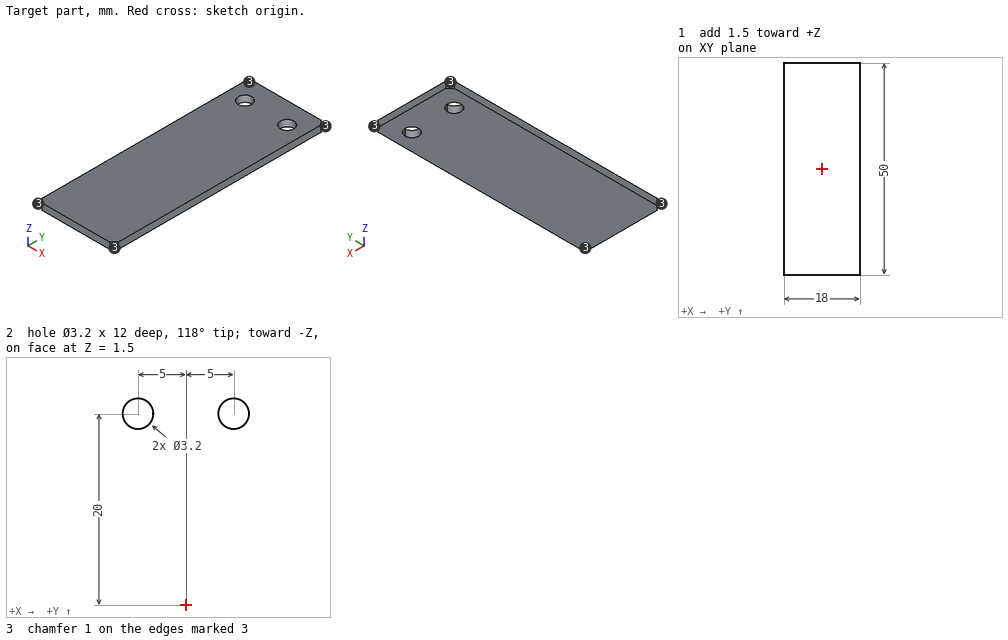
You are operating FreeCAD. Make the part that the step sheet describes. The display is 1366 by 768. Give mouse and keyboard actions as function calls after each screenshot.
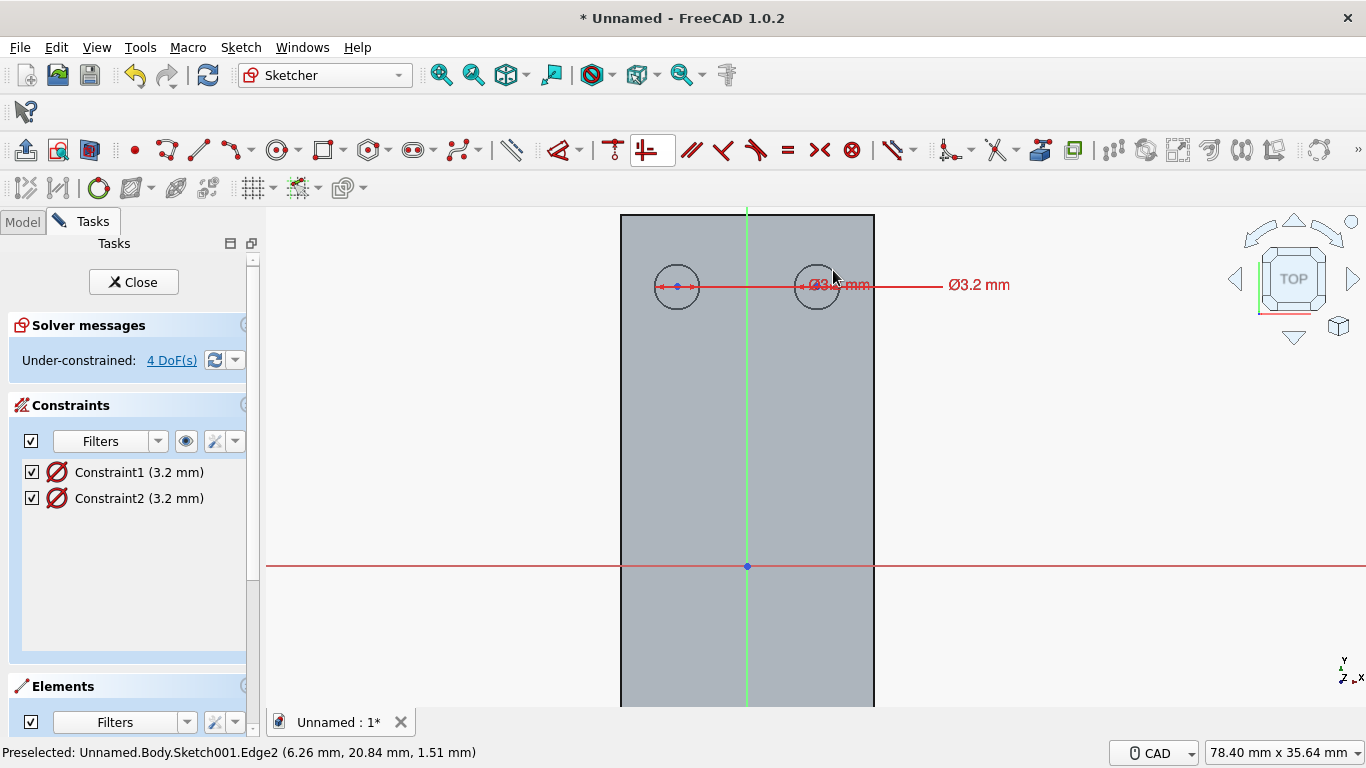
click(677, 287)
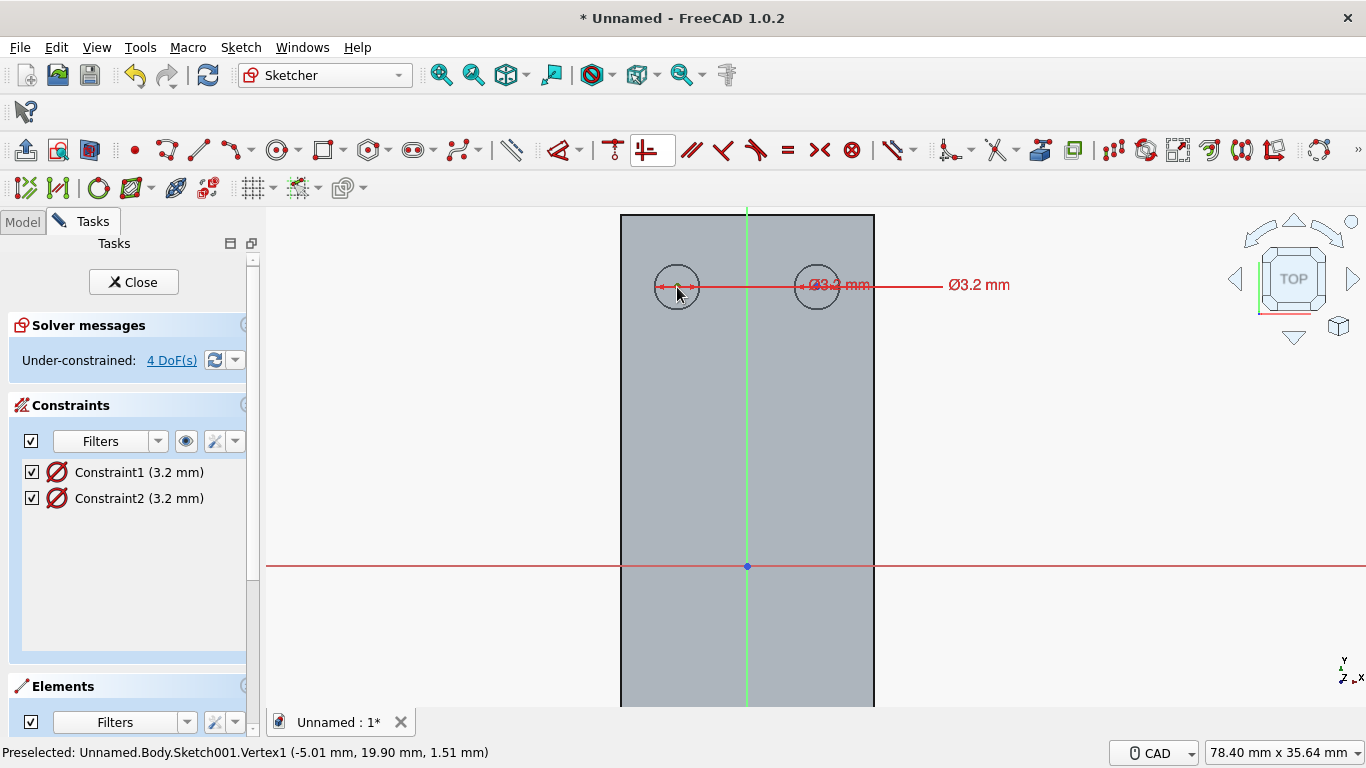
click(817, 287)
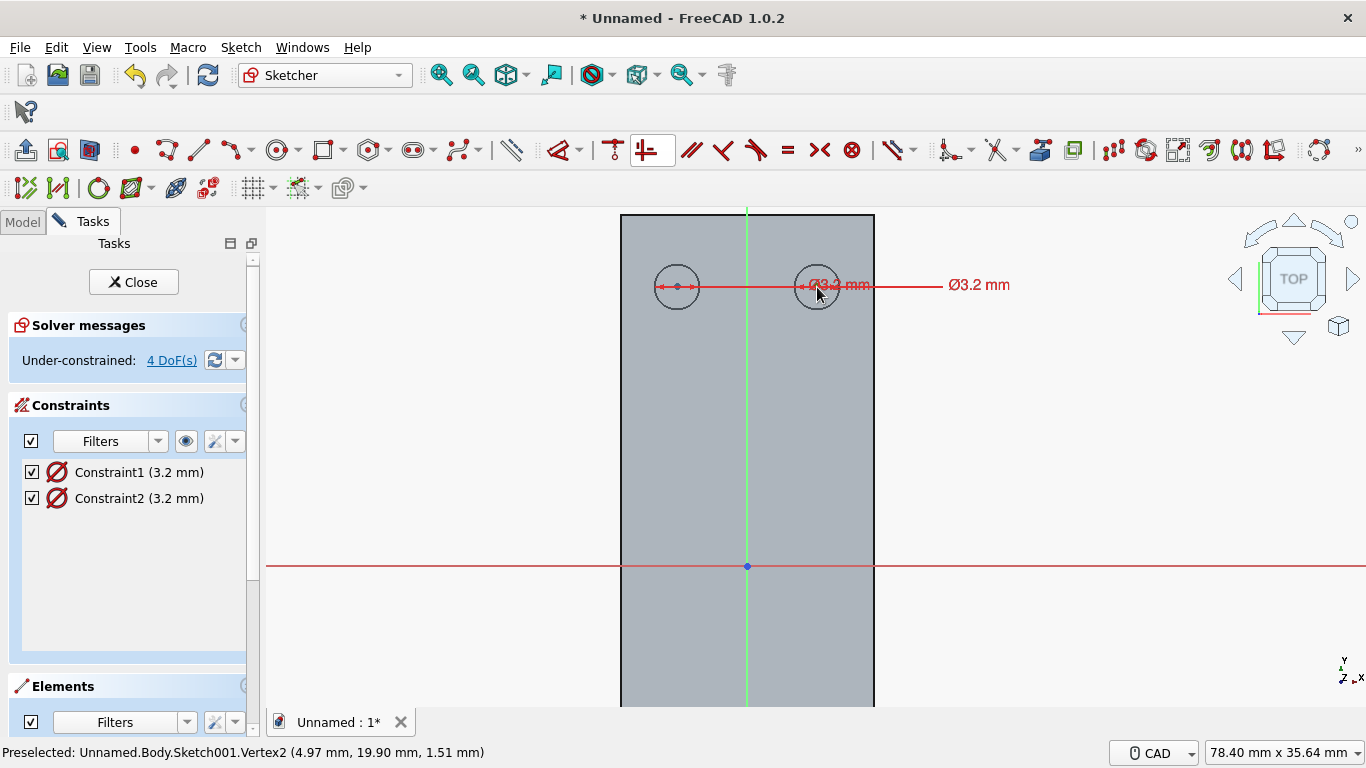
key(h)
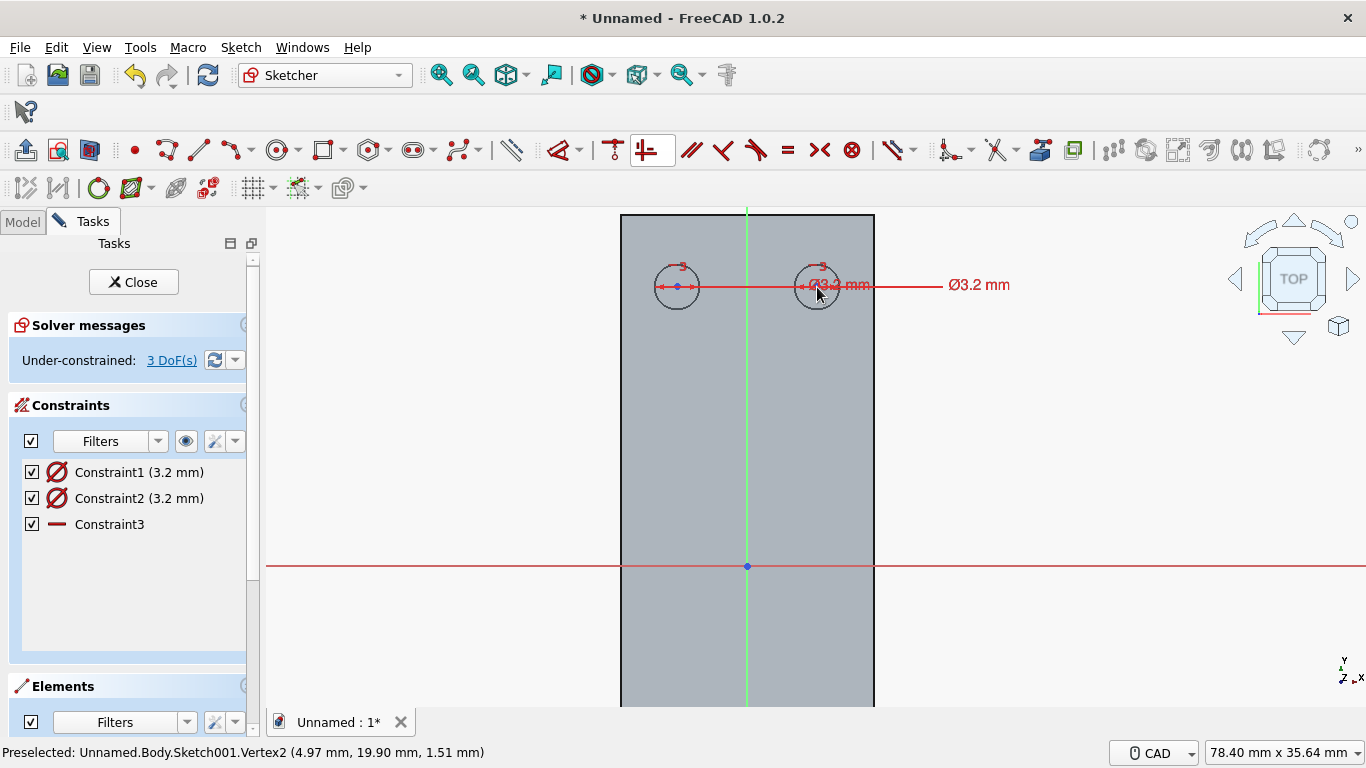
click(677, 287)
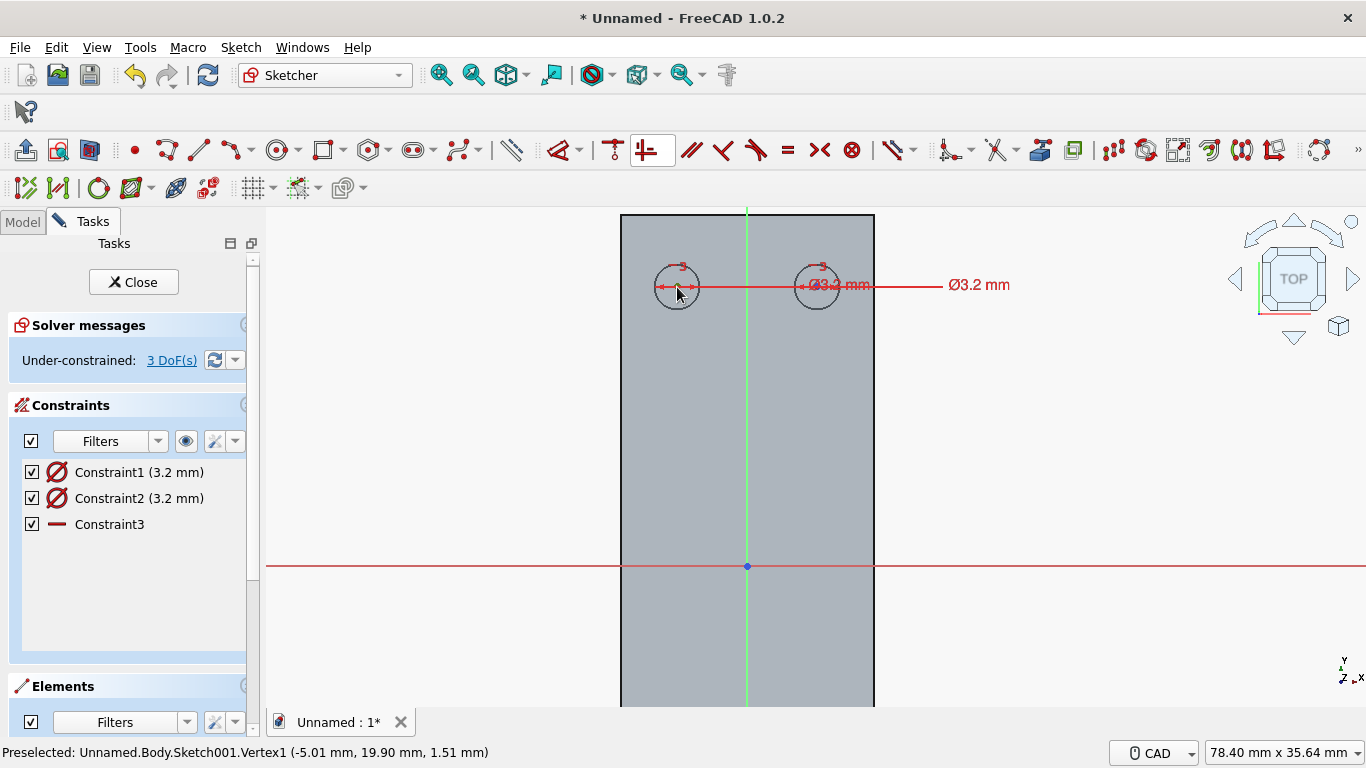
key(l)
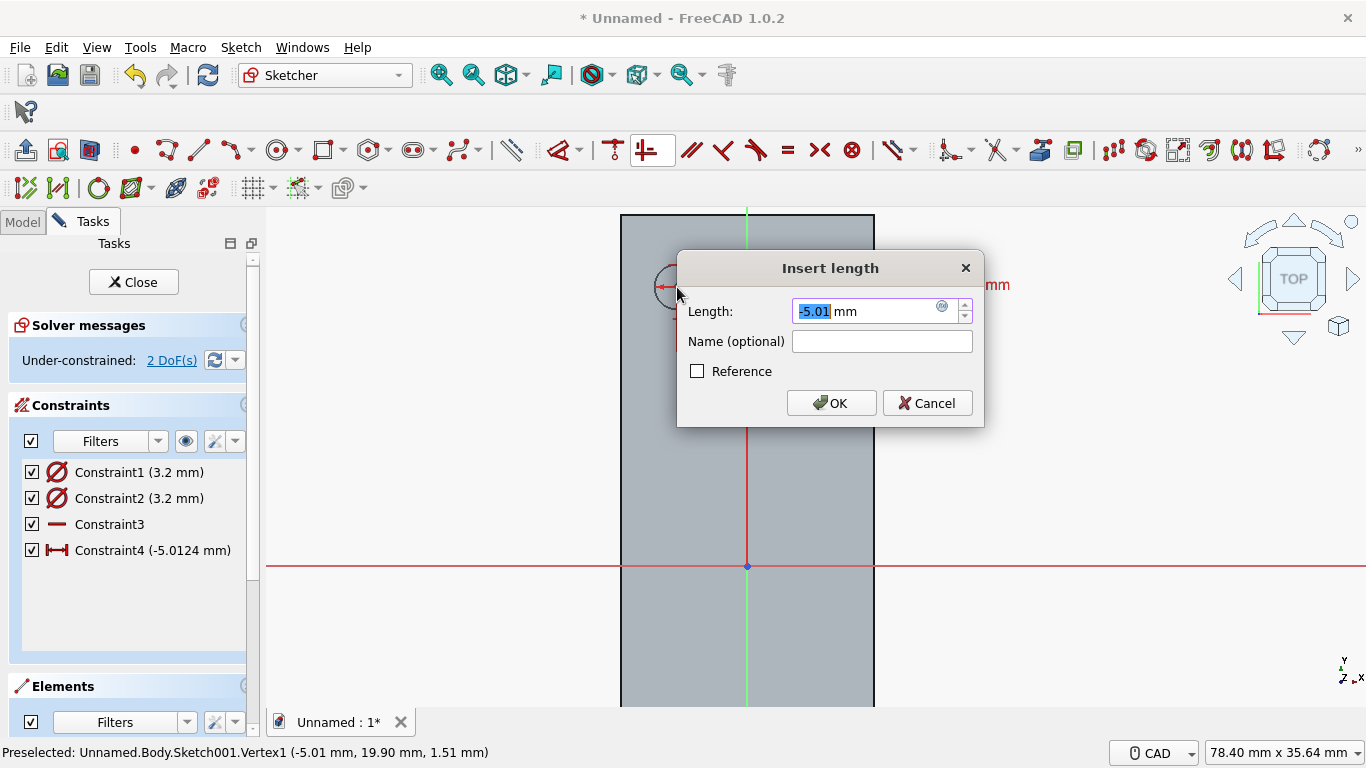
text(-5)
key(Return)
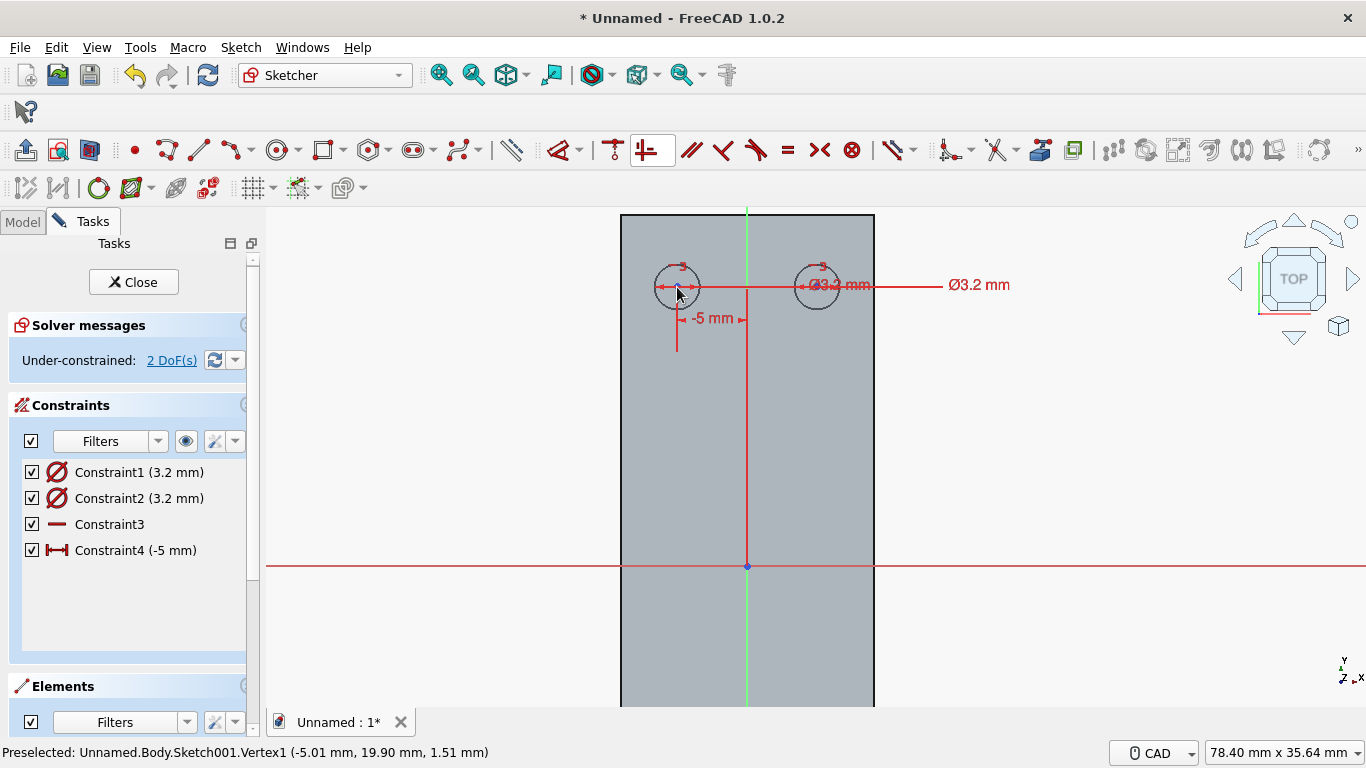
click(817, 287)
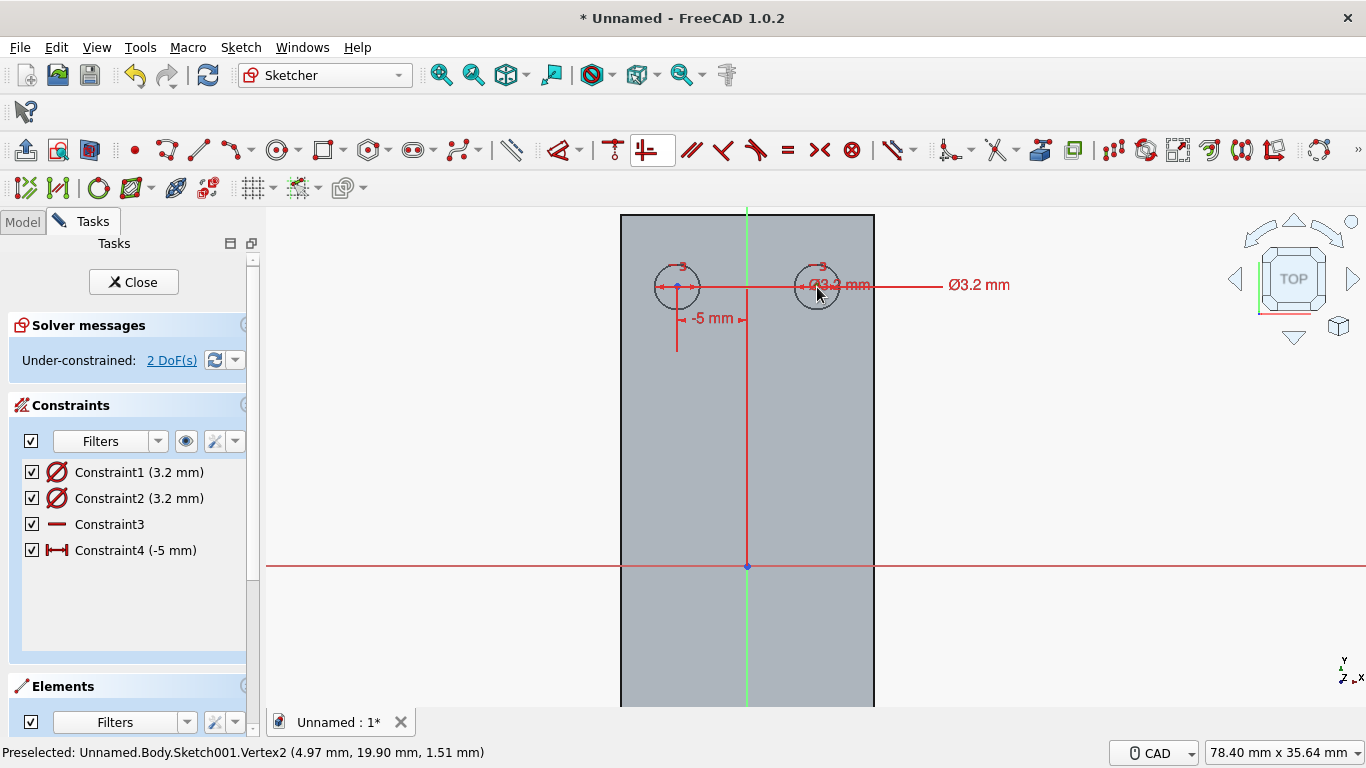
click(582, 150)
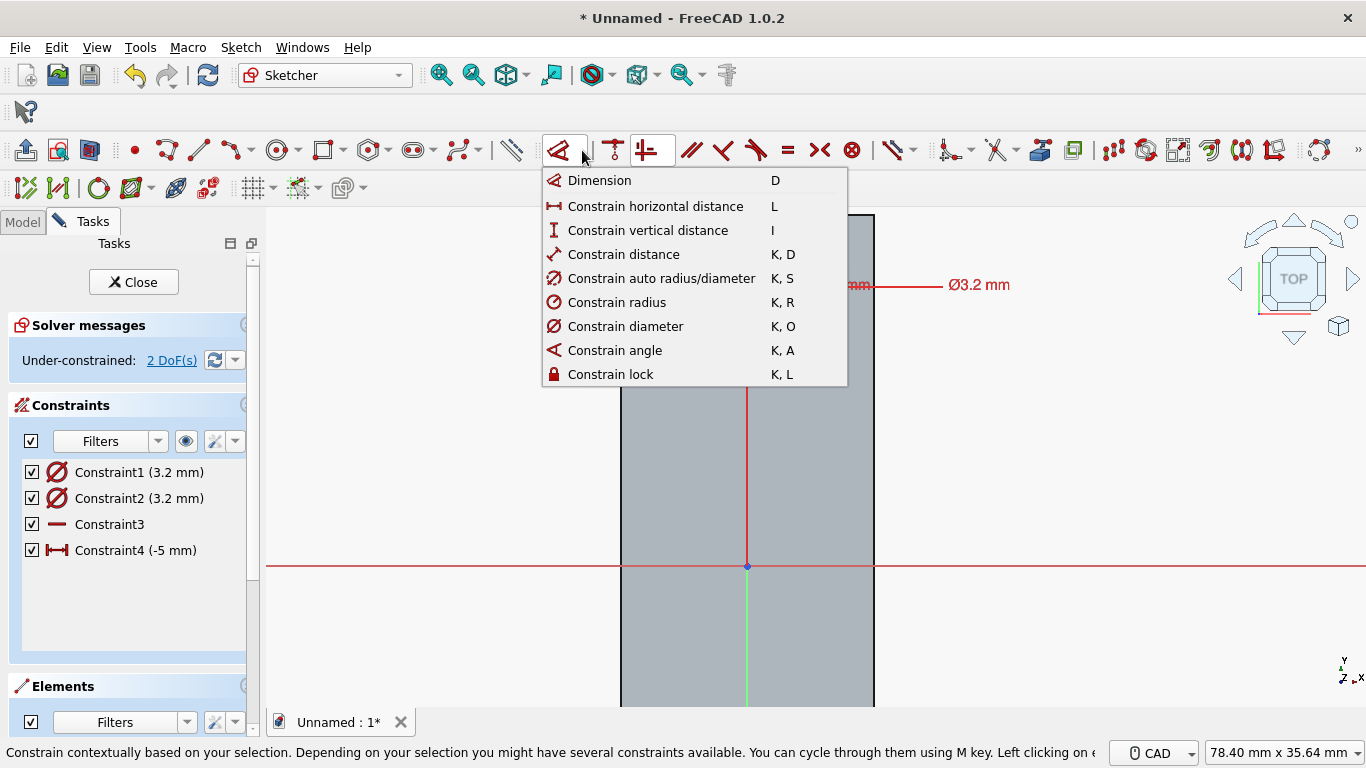
click(695, 206)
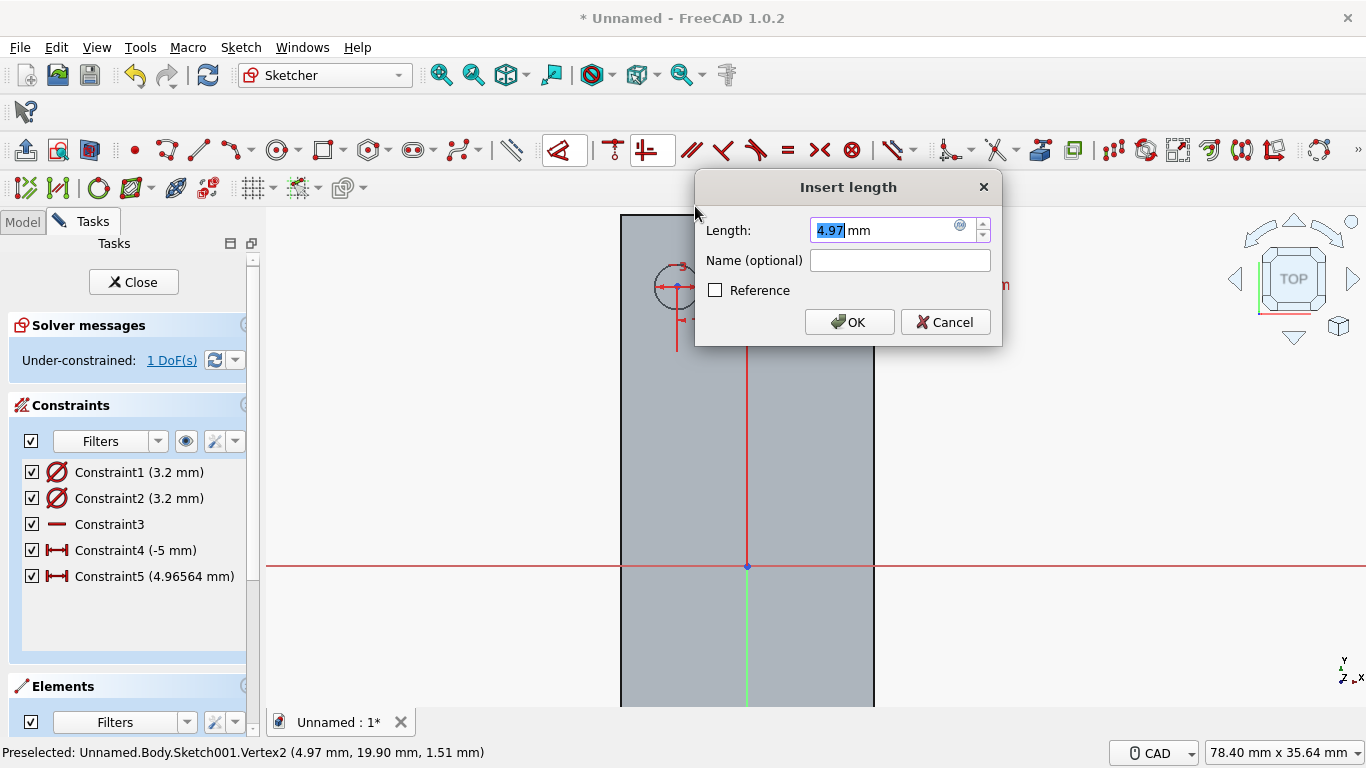
text(5)
key(Return)